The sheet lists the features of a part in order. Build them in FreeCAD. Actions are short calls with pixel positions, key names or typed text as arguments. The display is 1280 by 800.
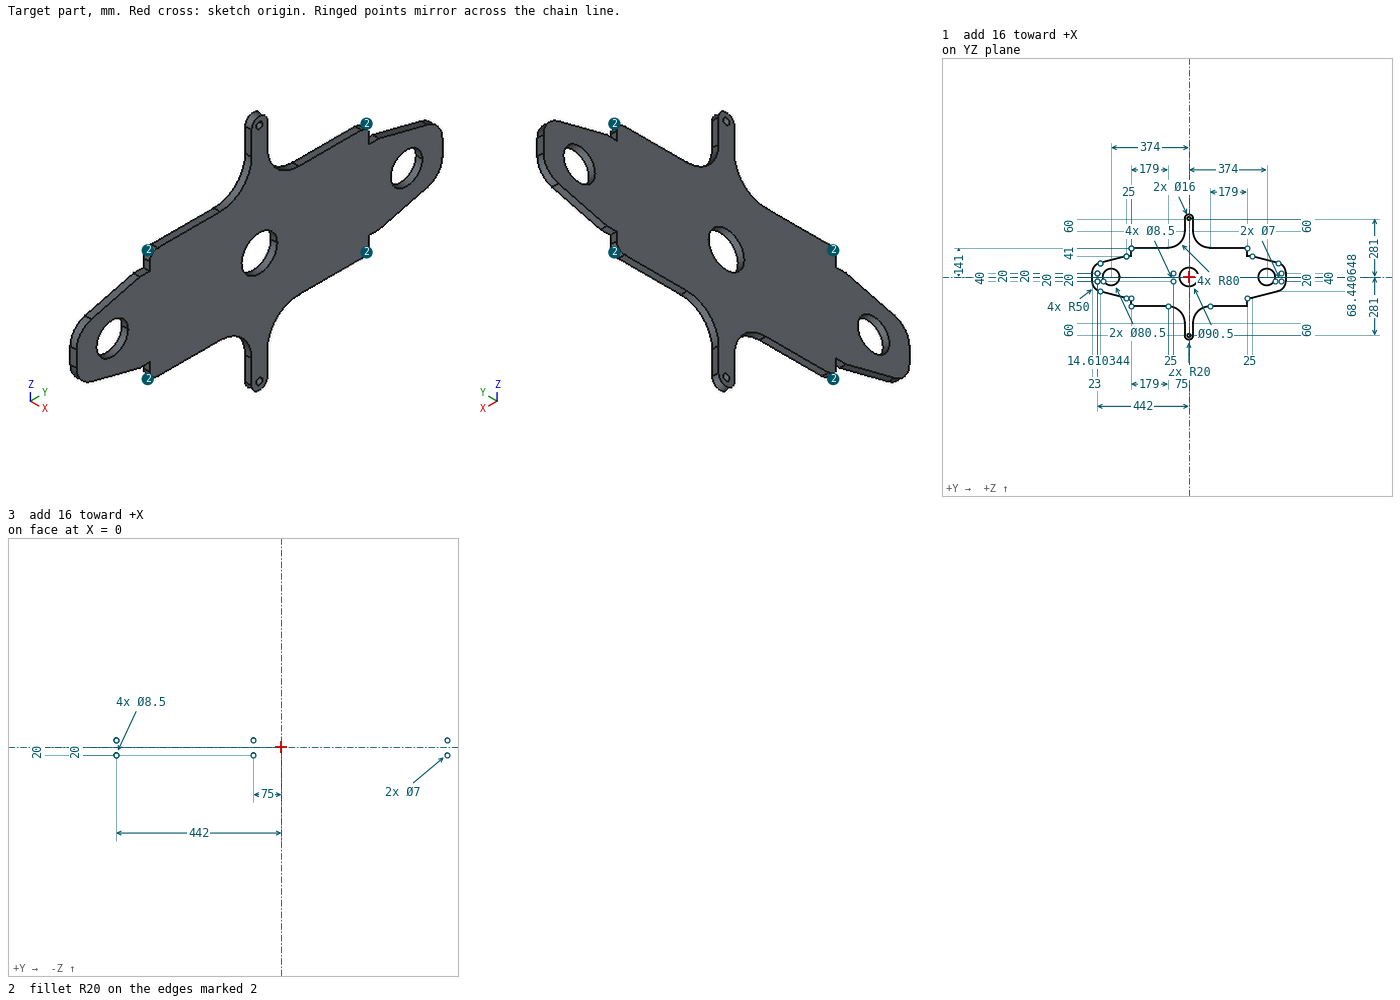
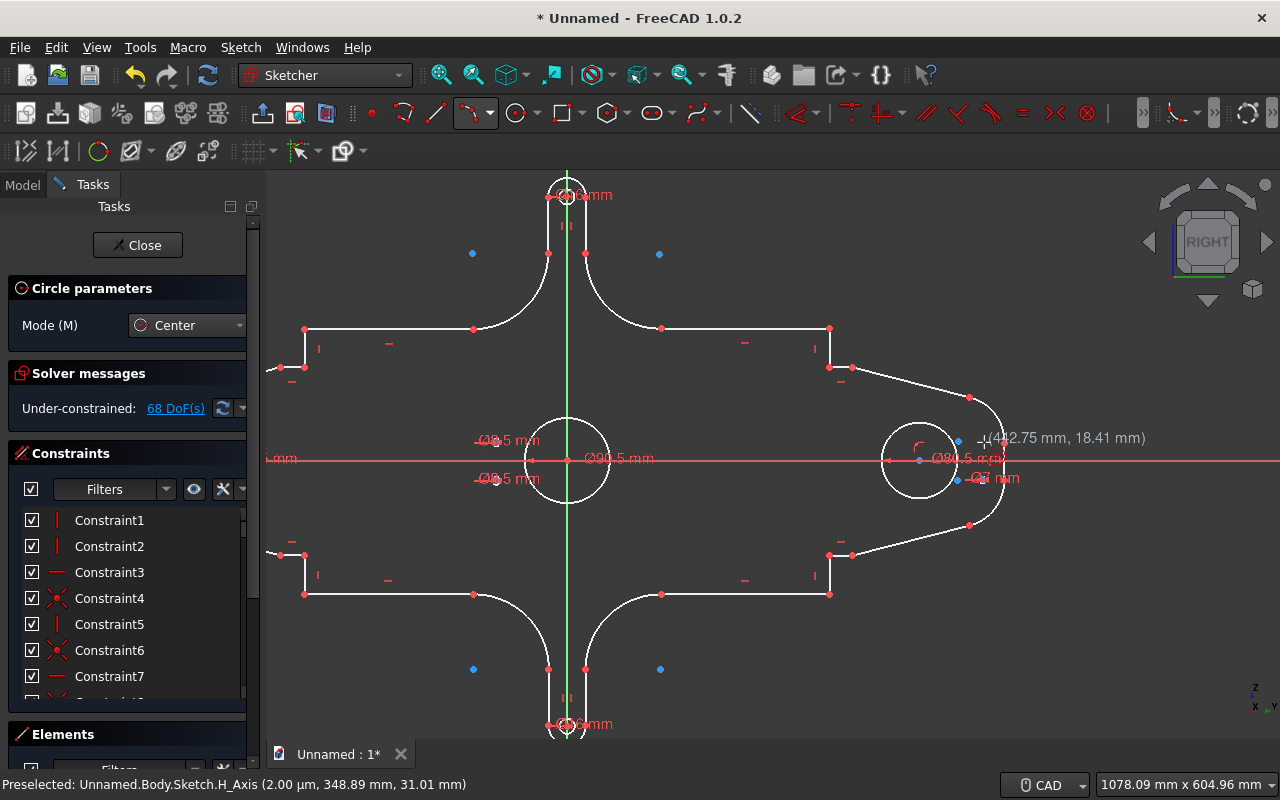
click(983, 442)
move(985, 439)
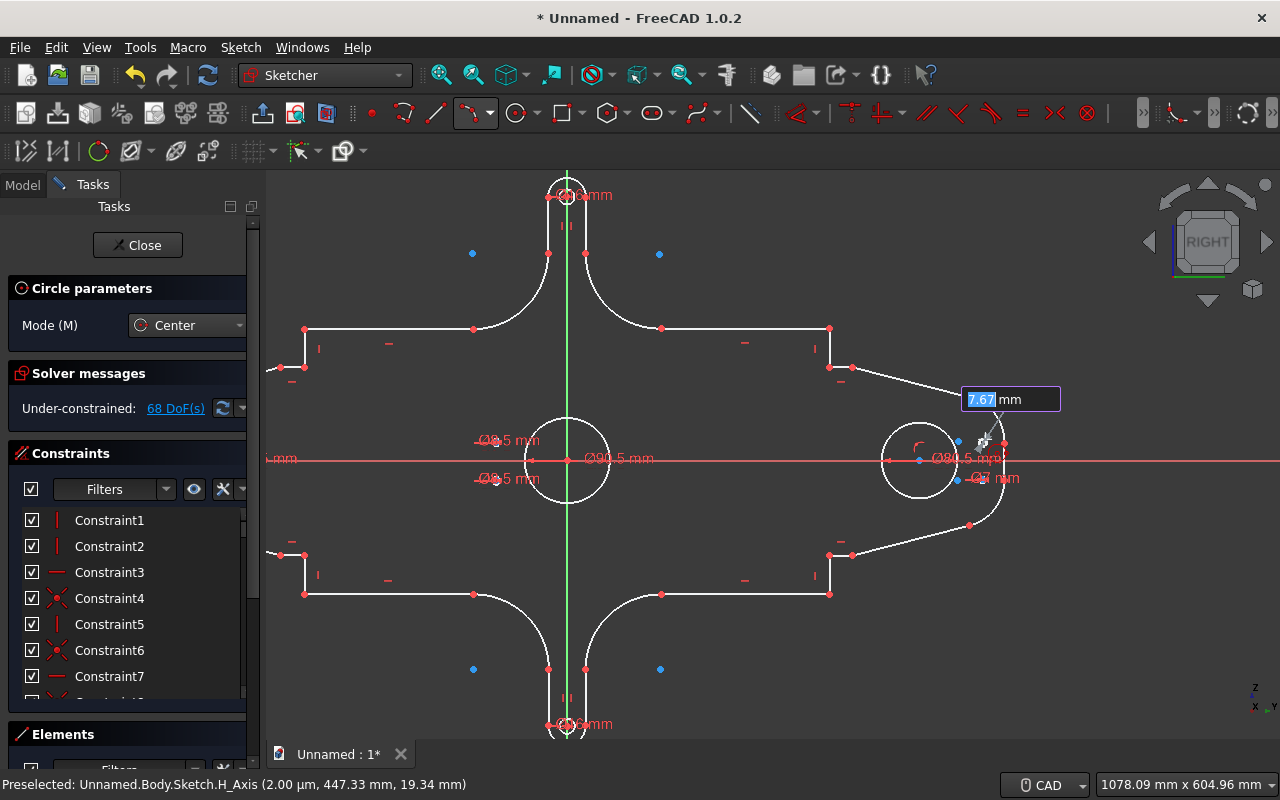
text(7)
key(Return)
key(Escape)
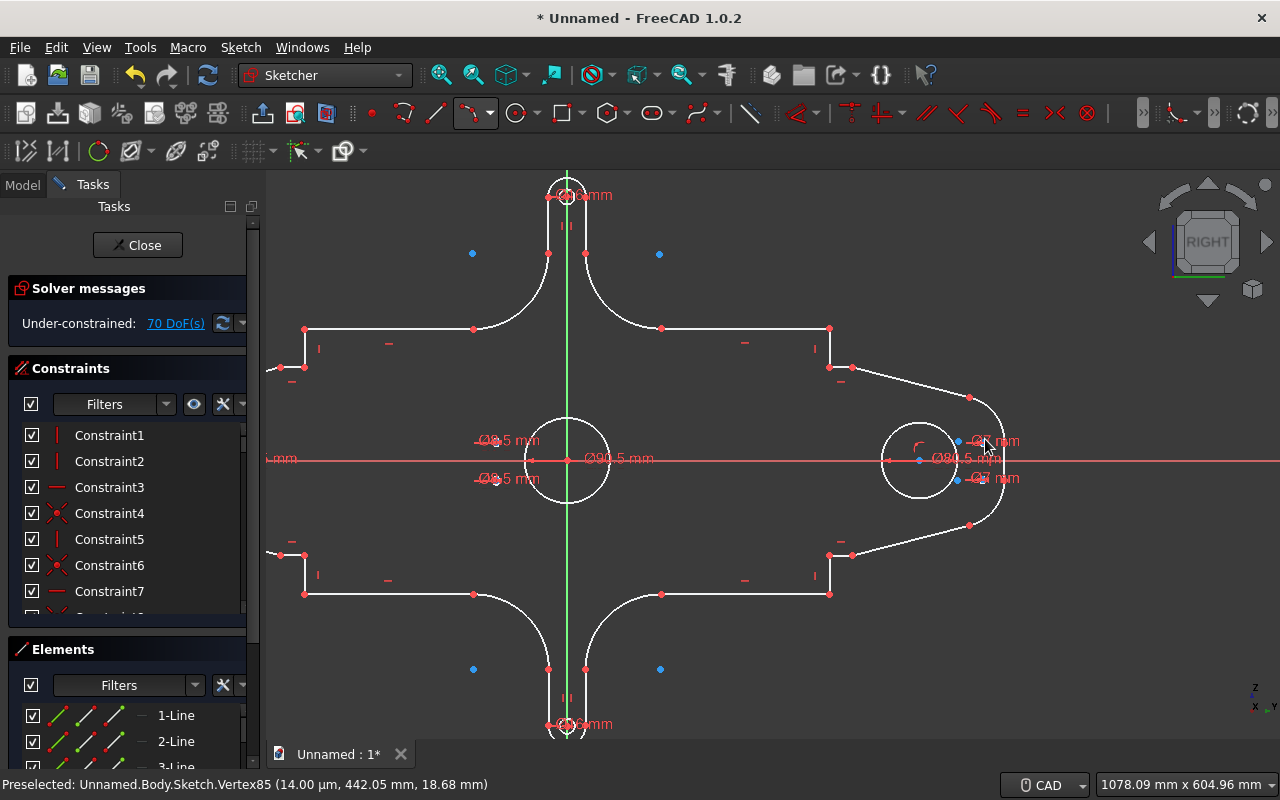
click(586, 237)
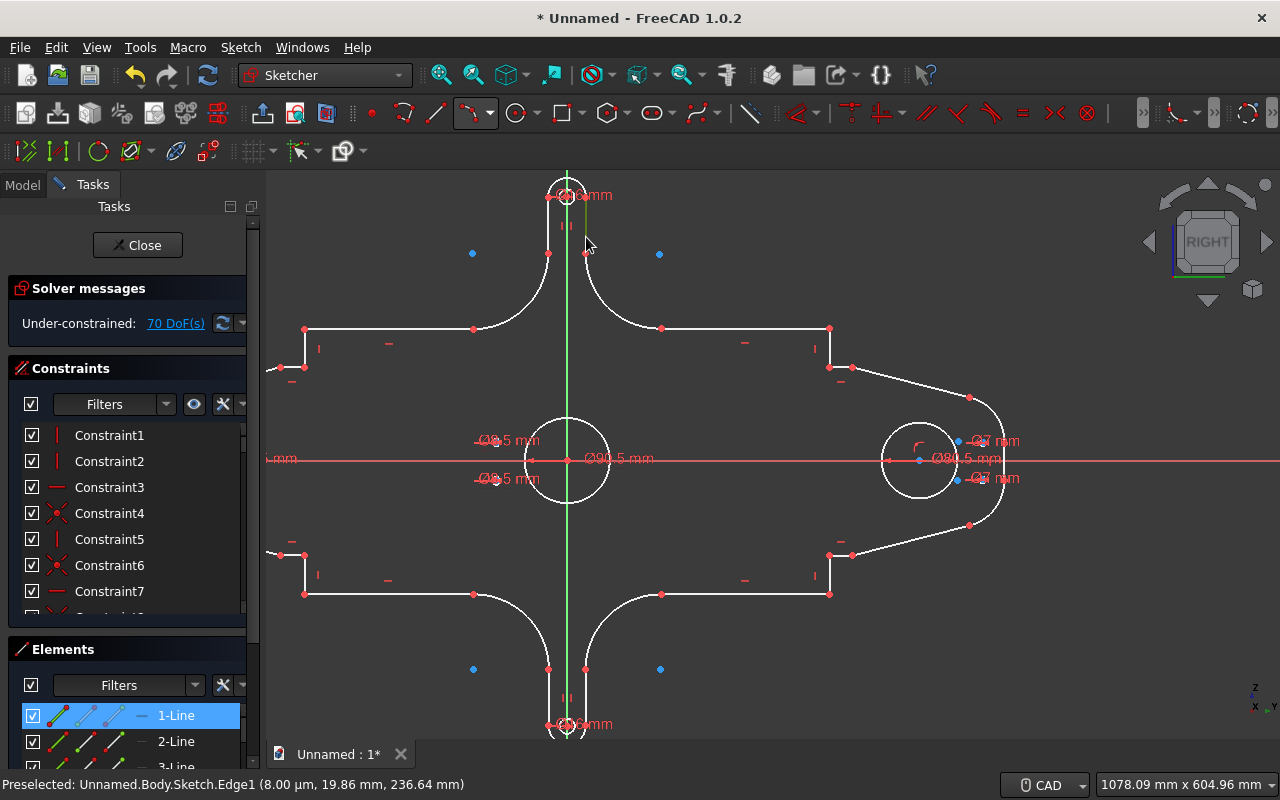
scroll(984, 442, down, 2)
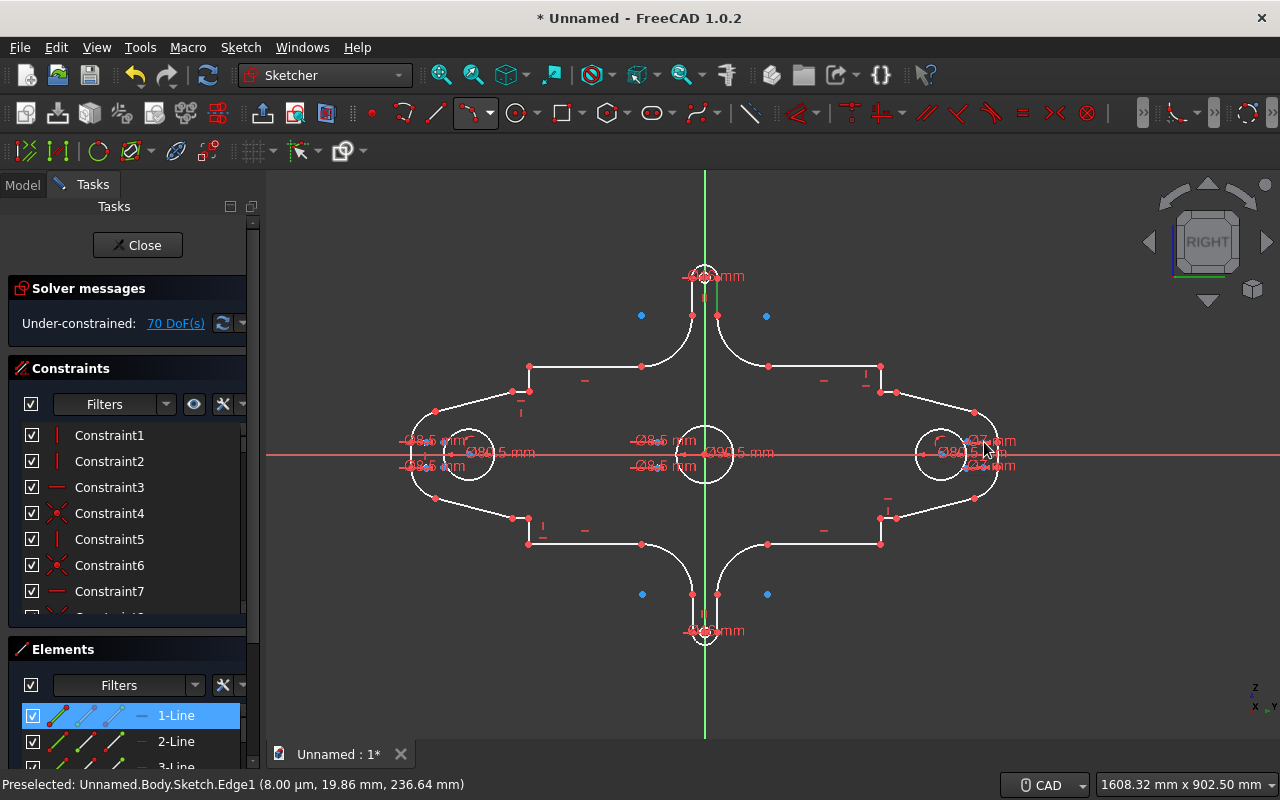
scroll(712, 268, up, 4)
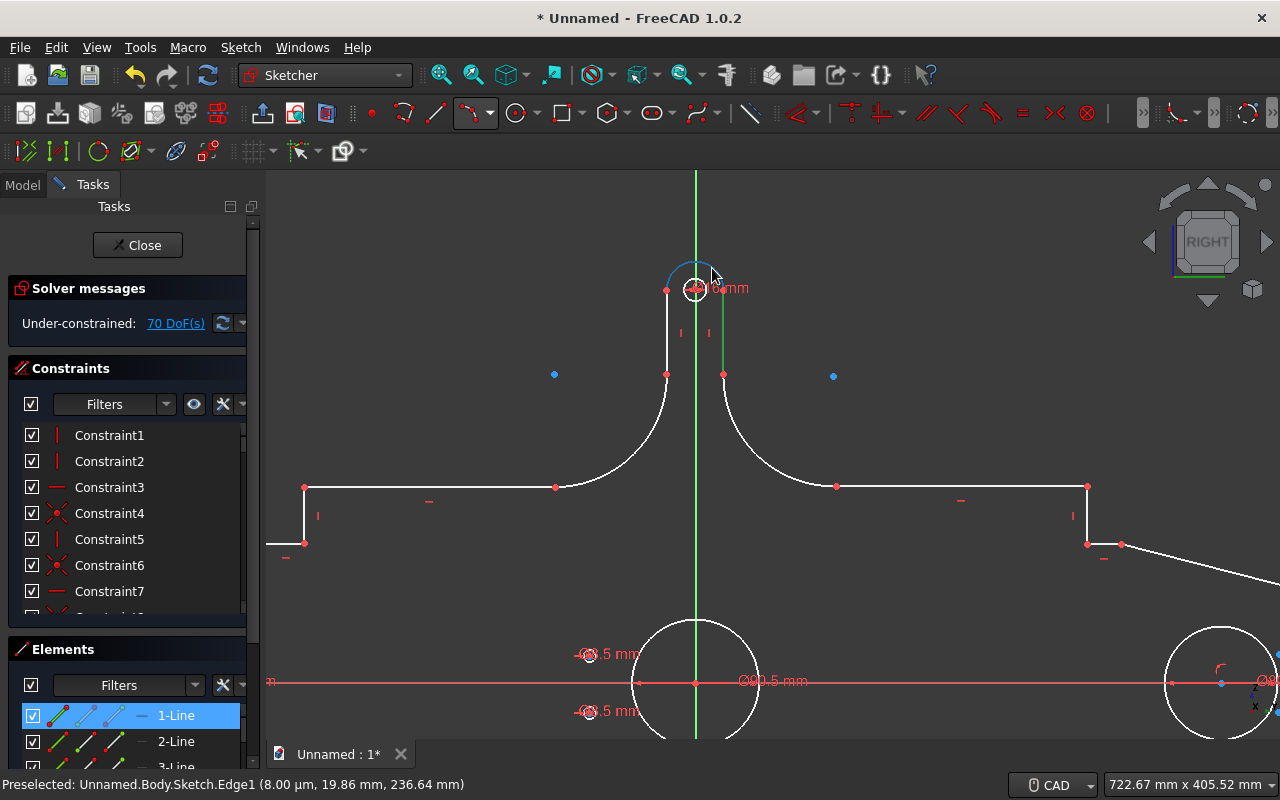
click(712, 267)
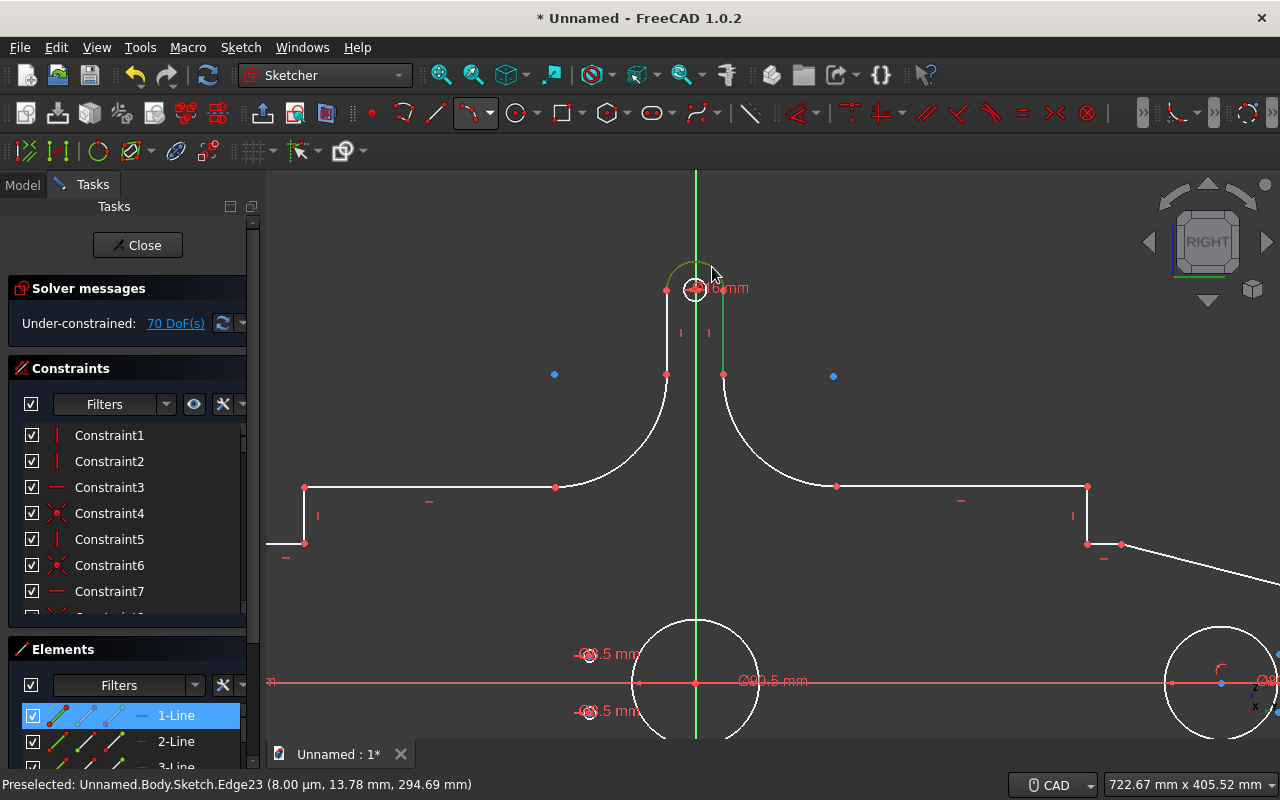
key(t)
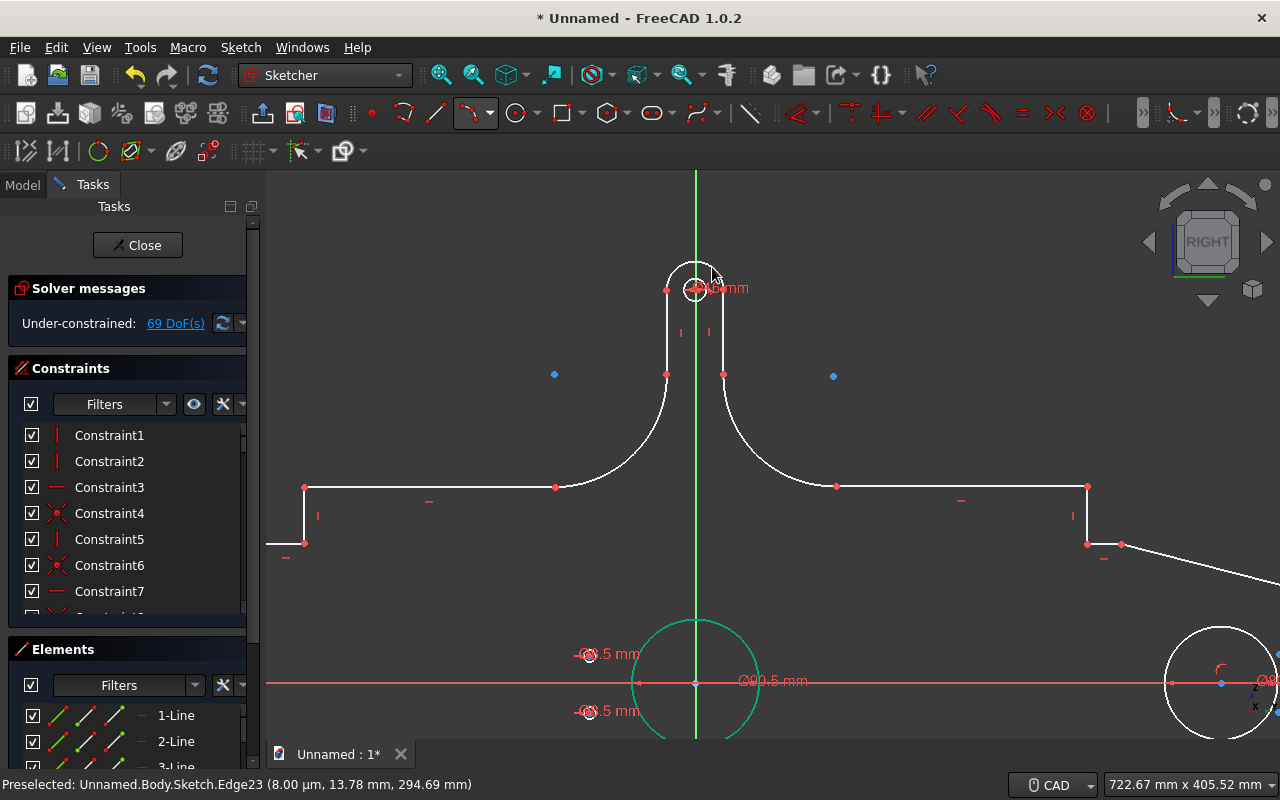
click(667, 316)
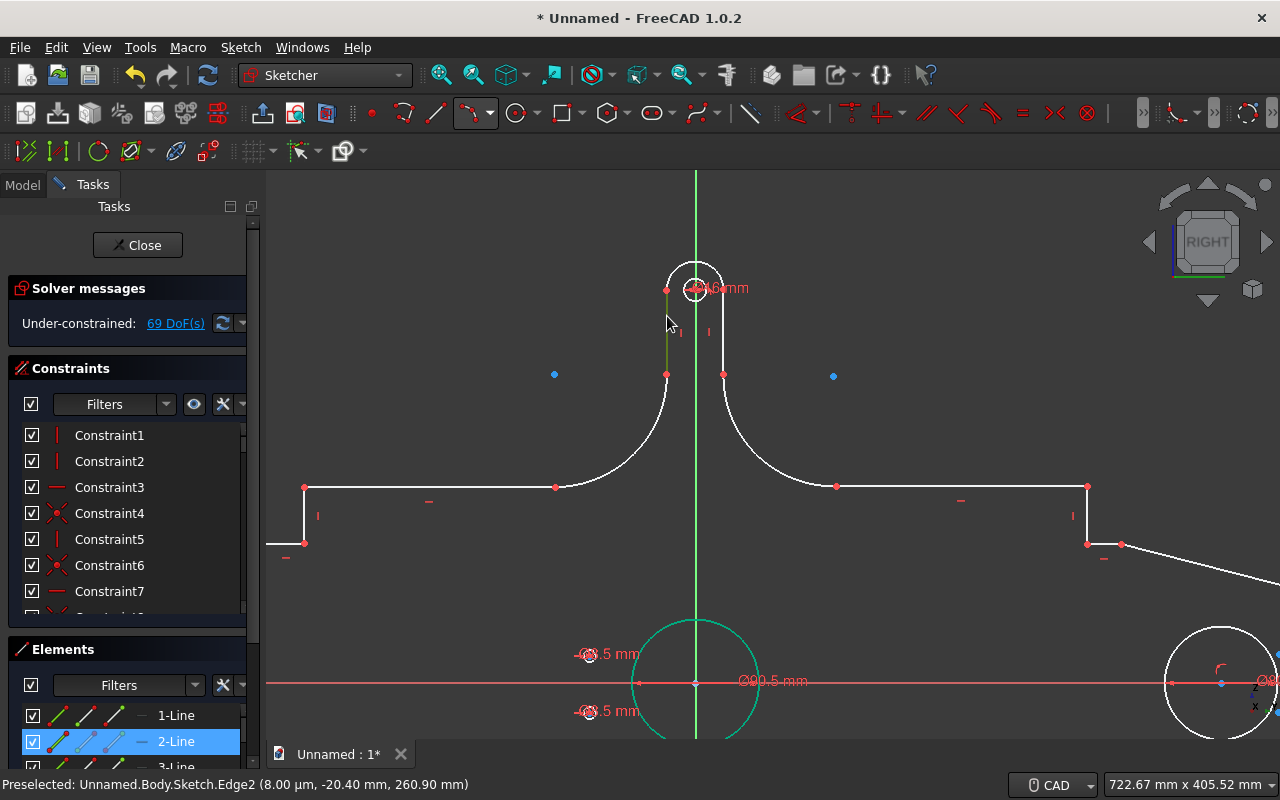
click(712, 267)